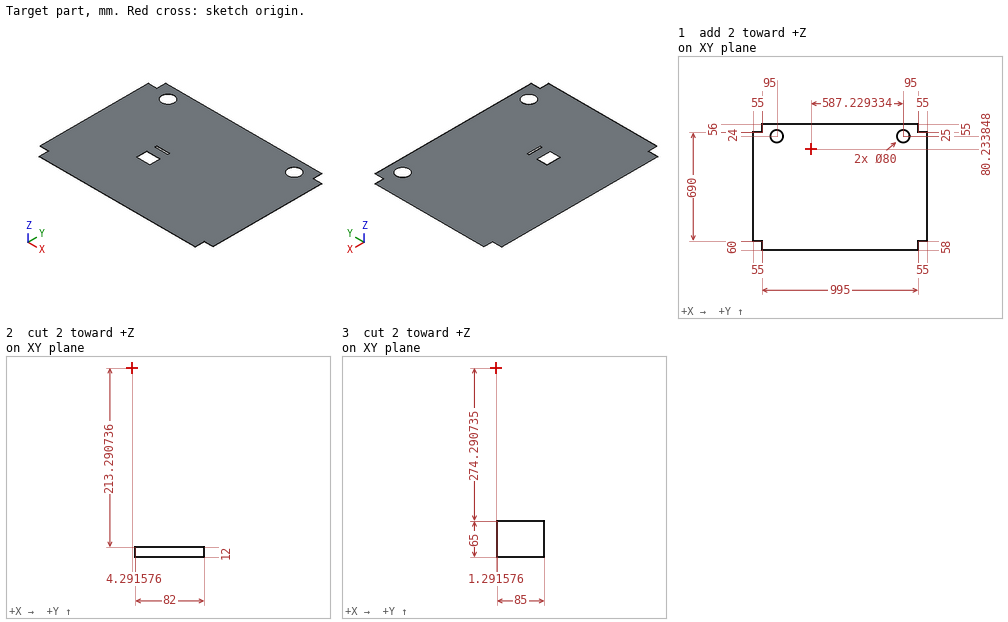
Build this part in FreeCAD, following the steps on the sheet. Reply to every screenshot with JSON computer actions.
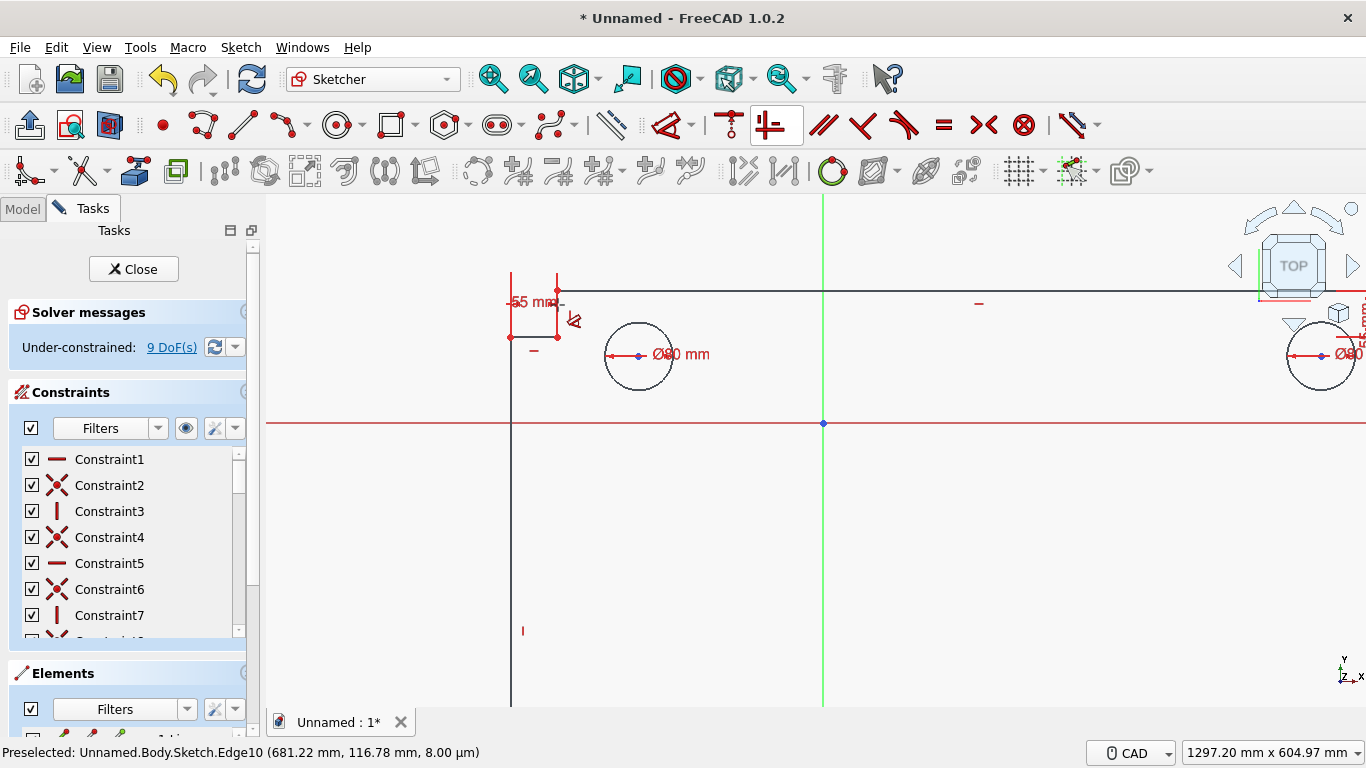
{"action": "left_click", "coordinate": [557, 305]}
{"action": "left_click", "coordinate": [591, 325]}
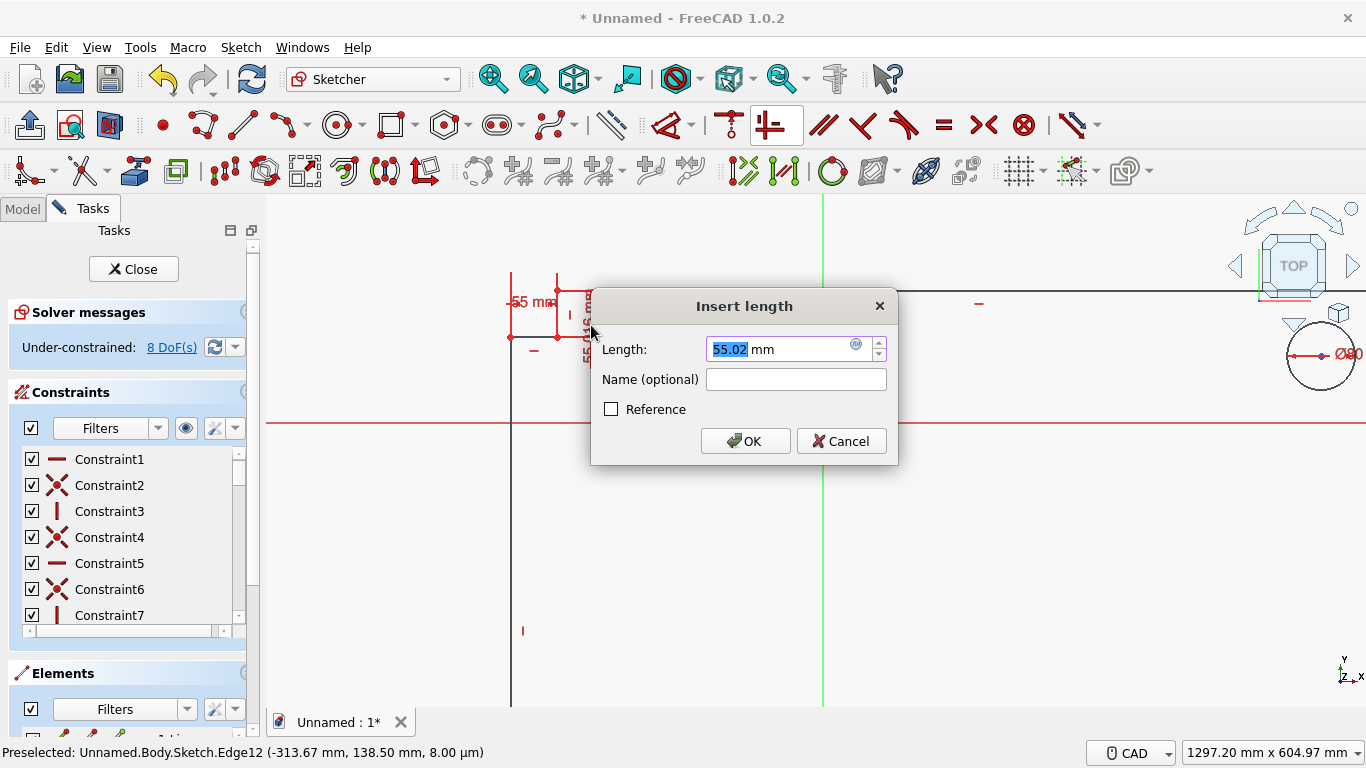
{"action": "type", "text": "56"}
{"action": "key", "text": "Return"}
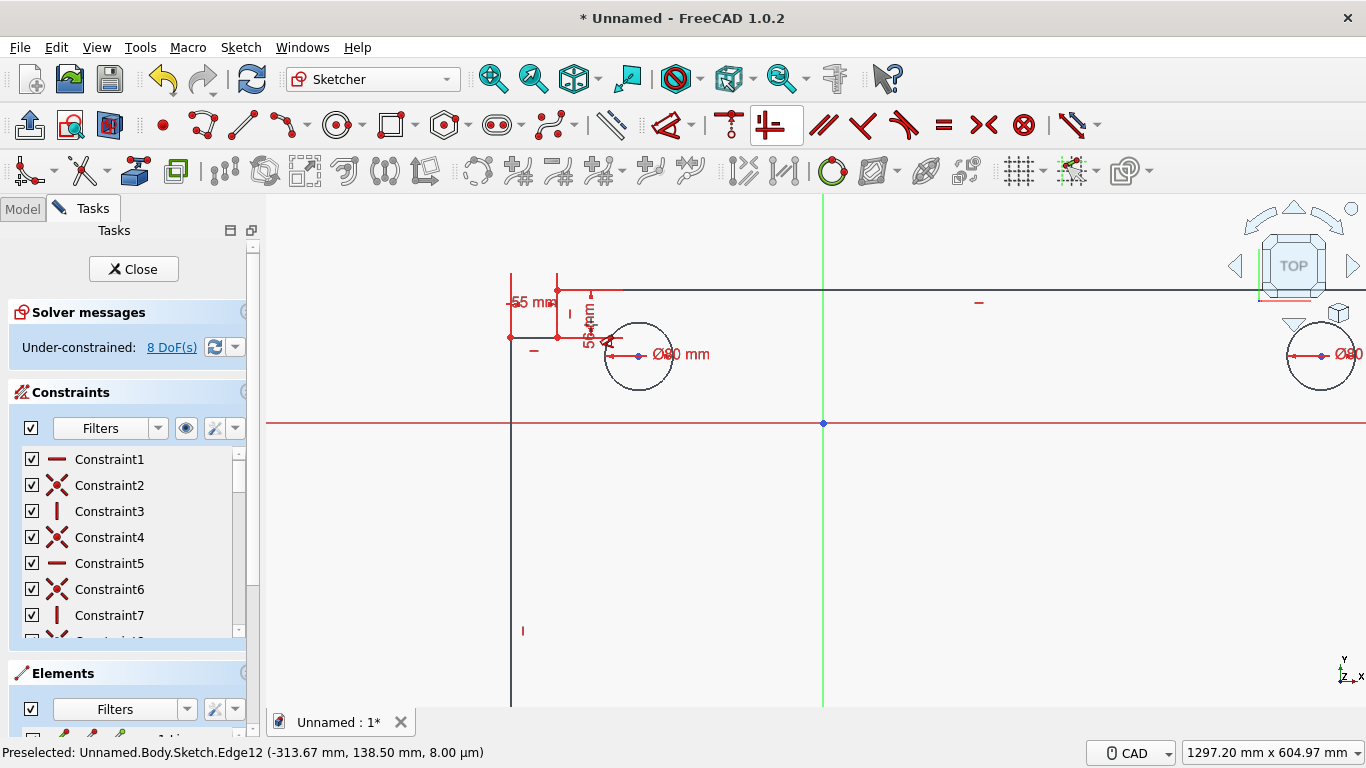
{"action": "left_click", "coordinate": [511, 513]}
{"action": "left_click", "coordinate": [477, 508]}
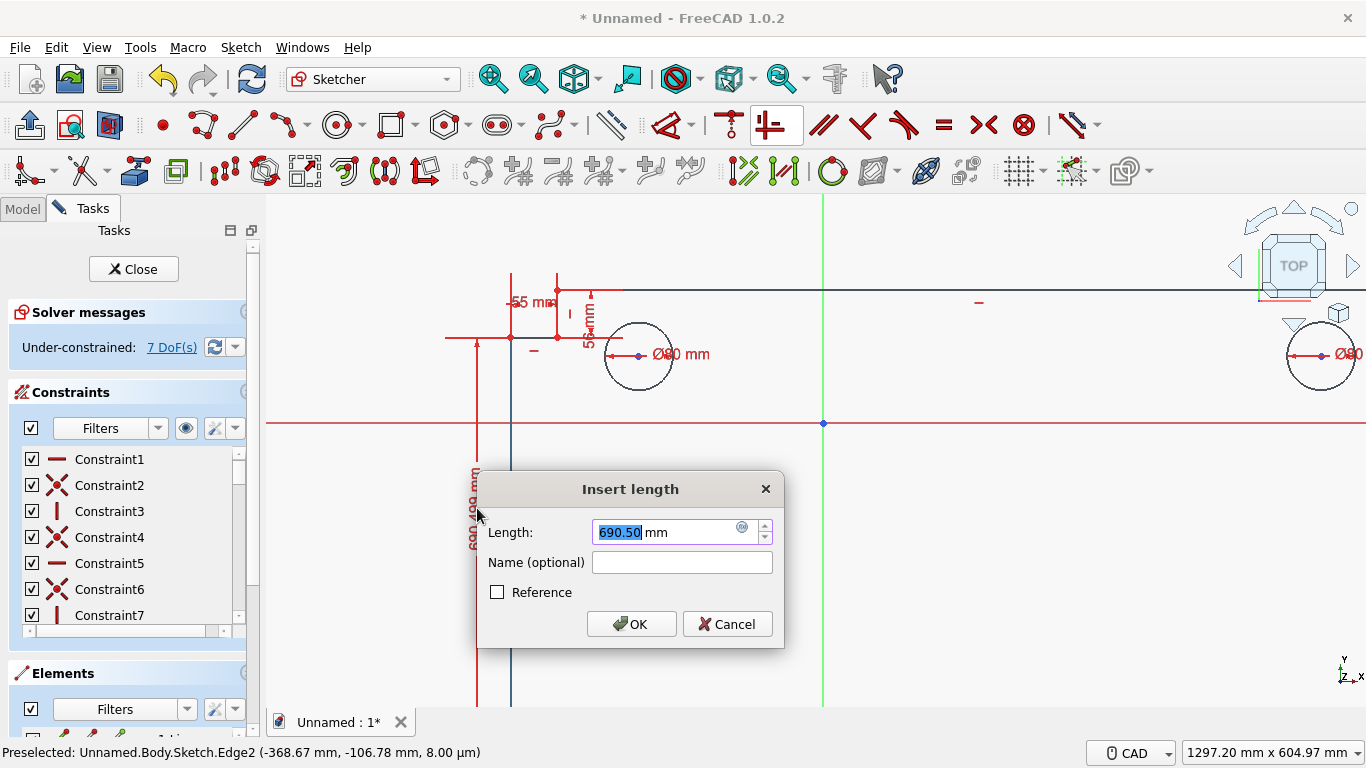
{"action": "type", "text": "690"}
{"action": "key", "text": "Return"}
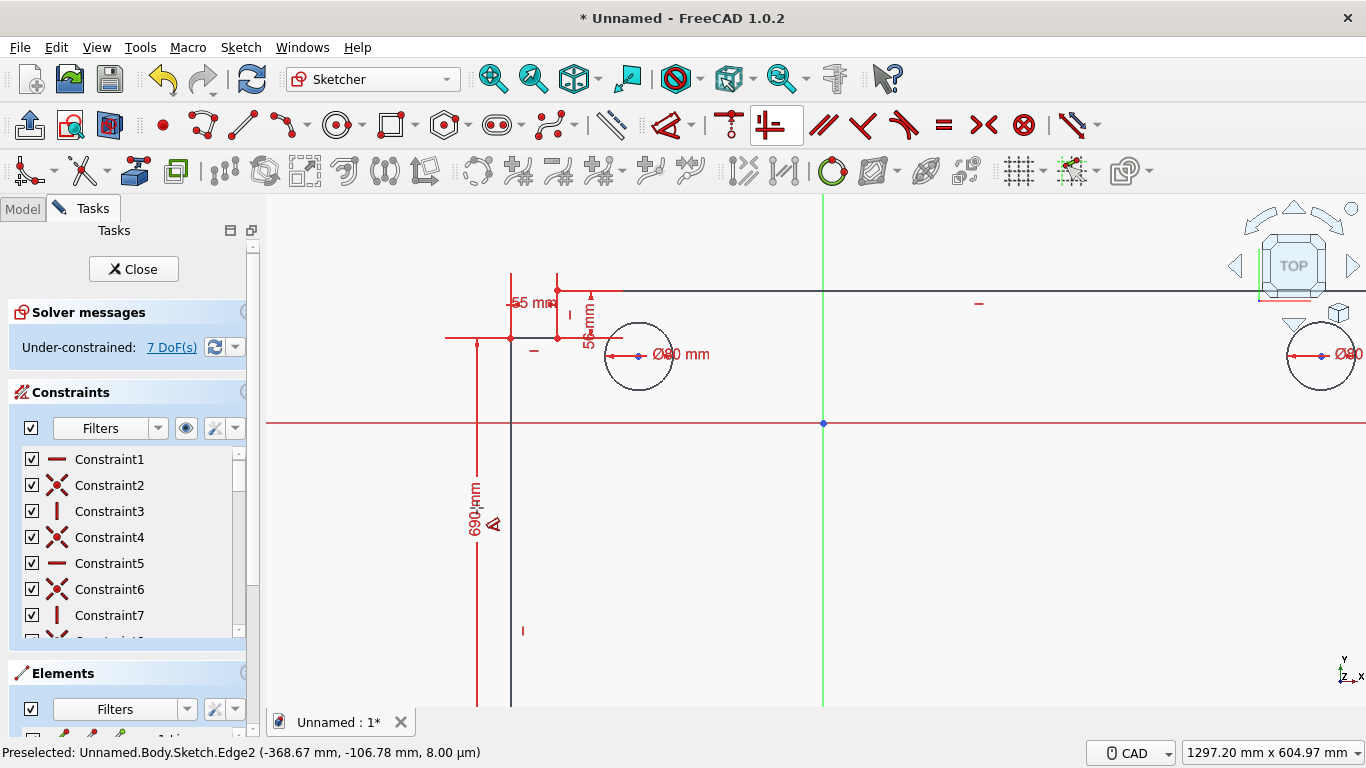
{"action": "scroll", "coordinate": [558, 305], "scroll_direction": "down", "scroll_amount": 4}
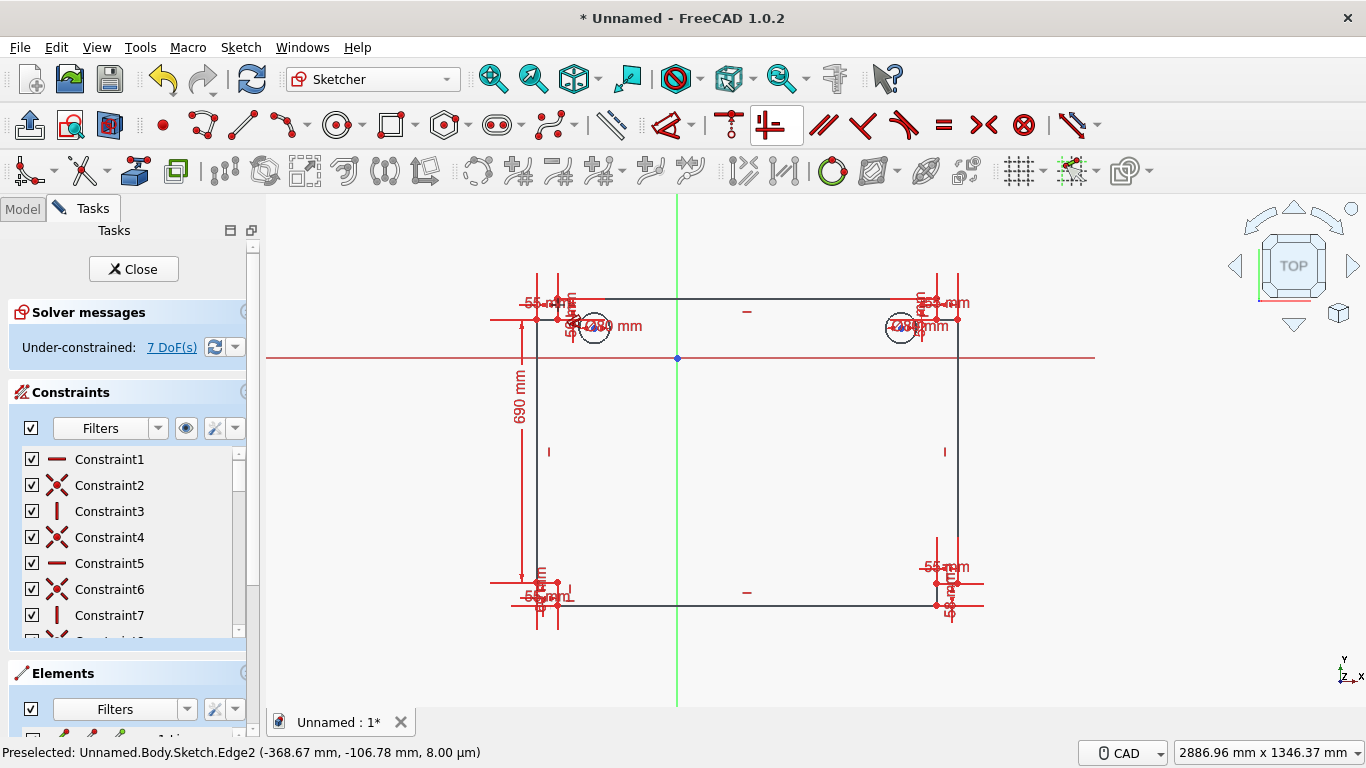
{"action": "scroll", "coordinate": [672, 606], "scroll_direction": "up", "scroll_amount": 5}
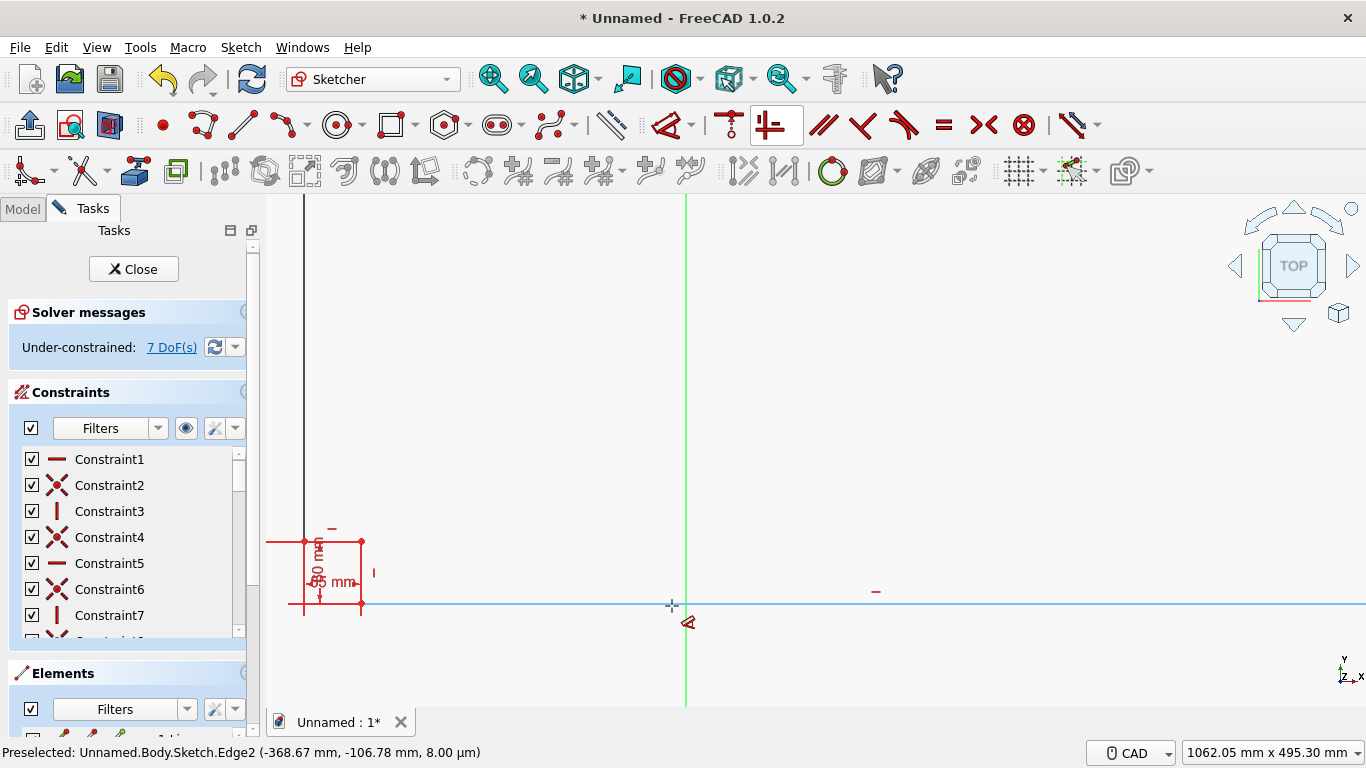
{"action": "left_click", "coordinate": [670, 604]}
{"action": "left_click", "coordinate": [781, 638]}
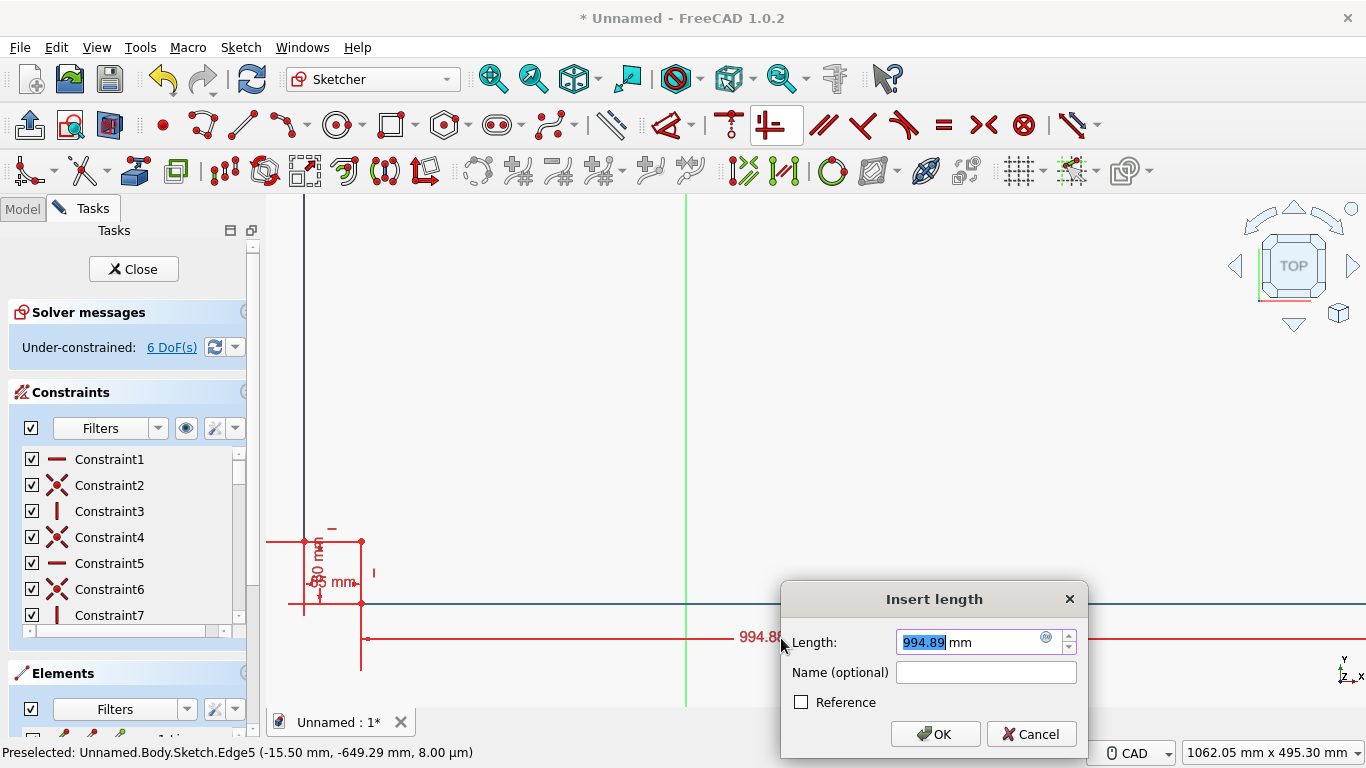
{"action": "type", "text": "995"}
{"action": "key", "text": "Return"}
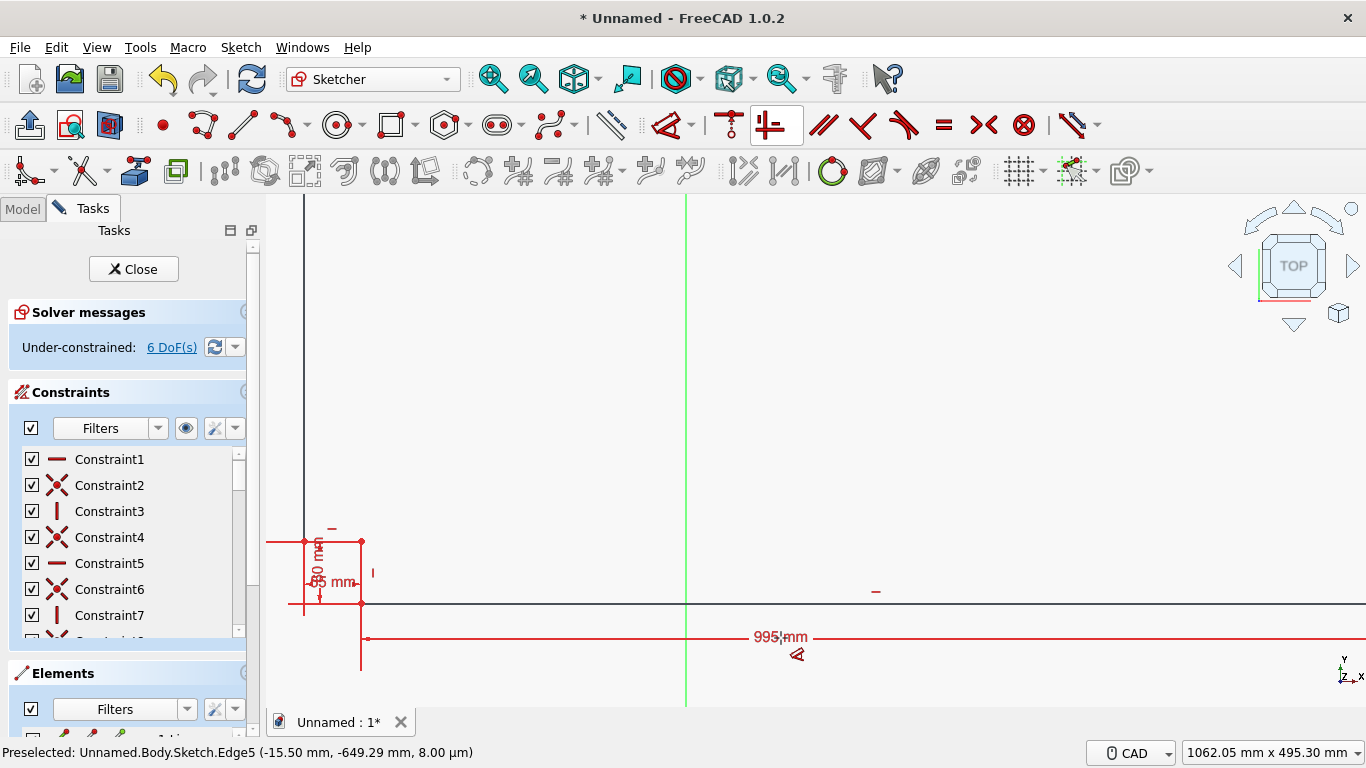
{"action": "scroll", "coordinate": [672, 606], "scroll_direction": "down", "scroll_amount": 5}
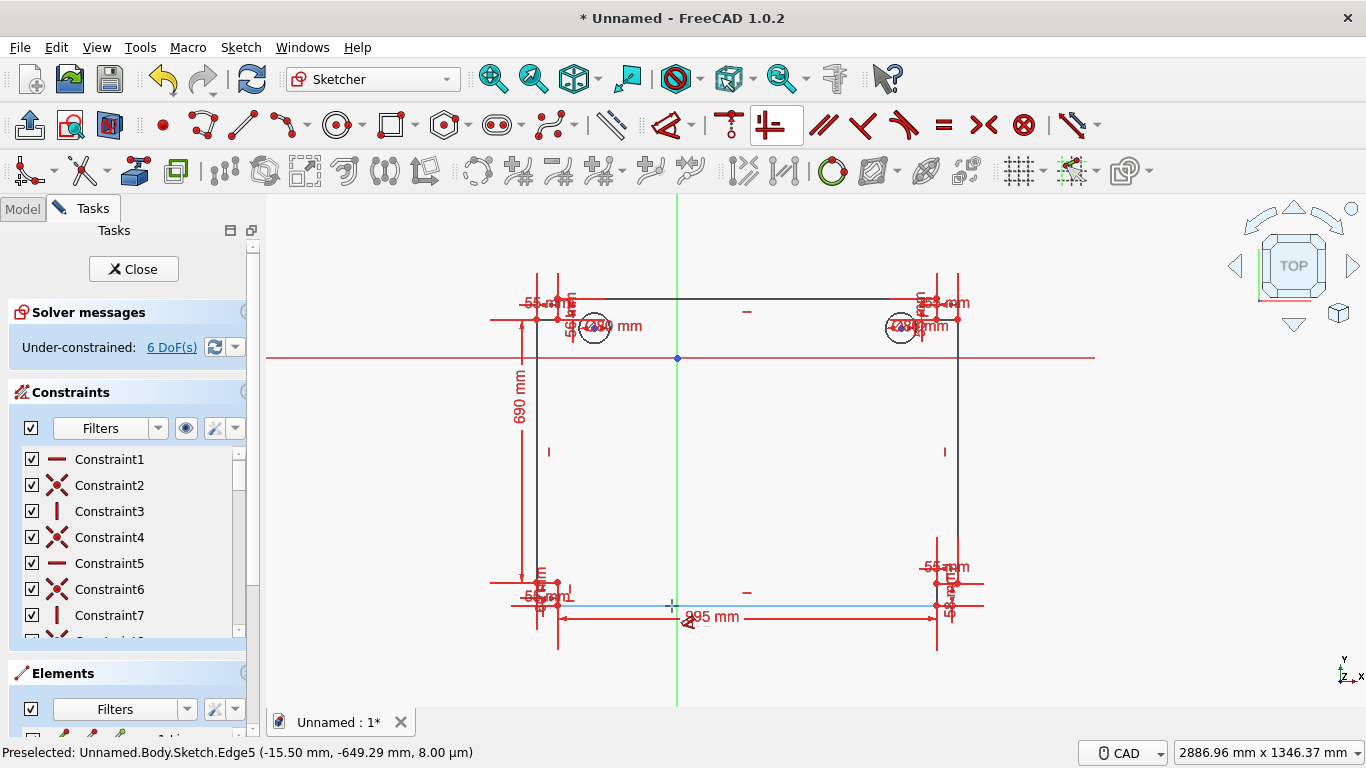
{"action": "left_click", "coordinate": [937, 320]}